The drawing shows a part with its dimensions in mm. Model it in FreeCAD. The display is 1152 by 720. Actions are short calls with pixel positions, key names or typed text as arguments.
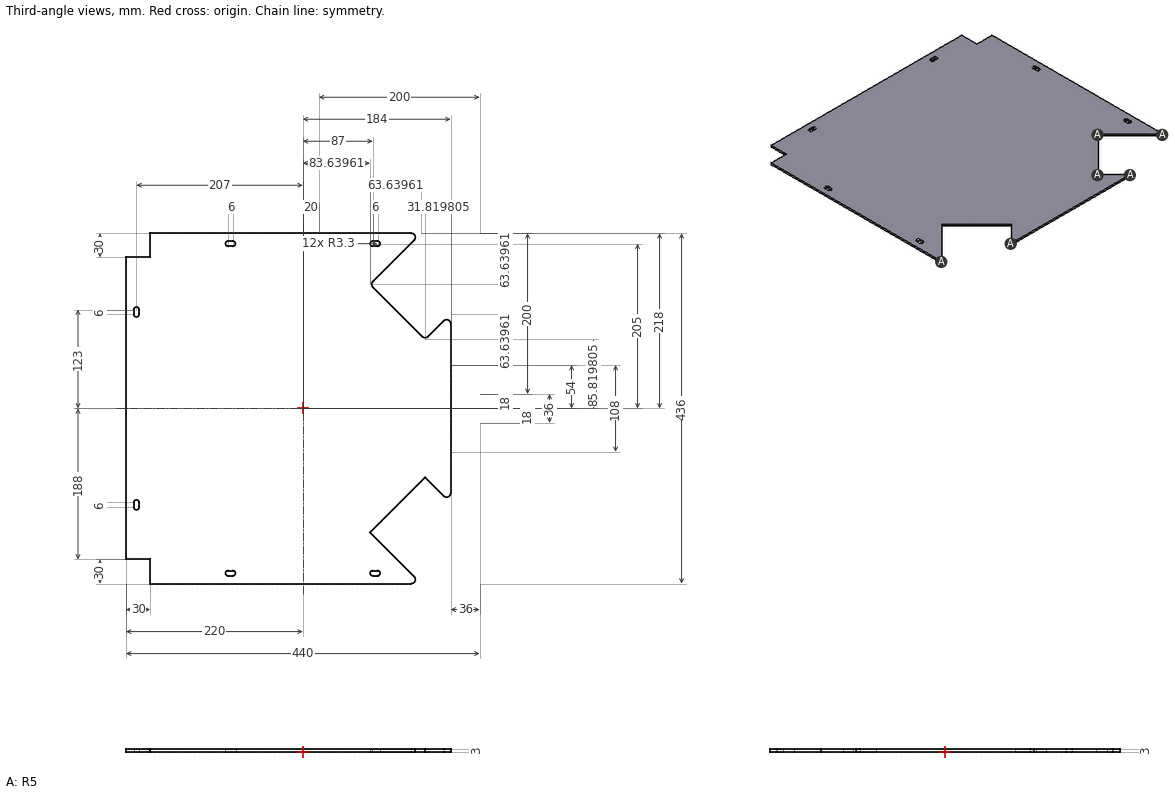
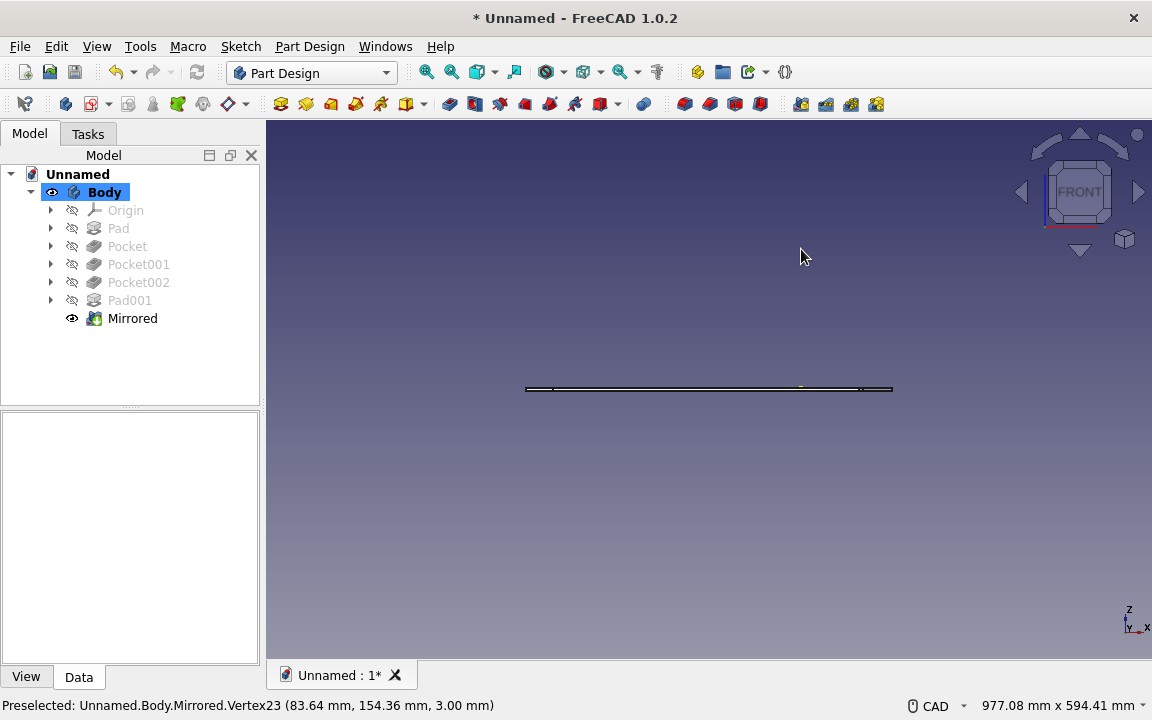
key(v)
key(f)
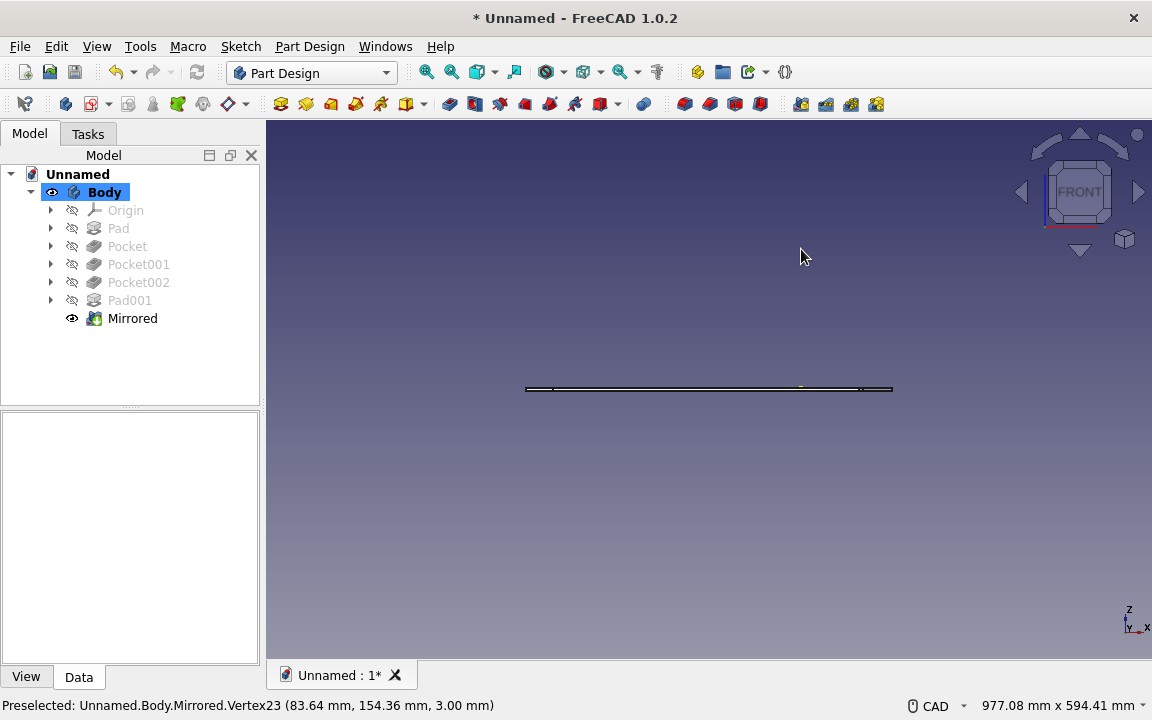
scroll(801, 389, up, 14)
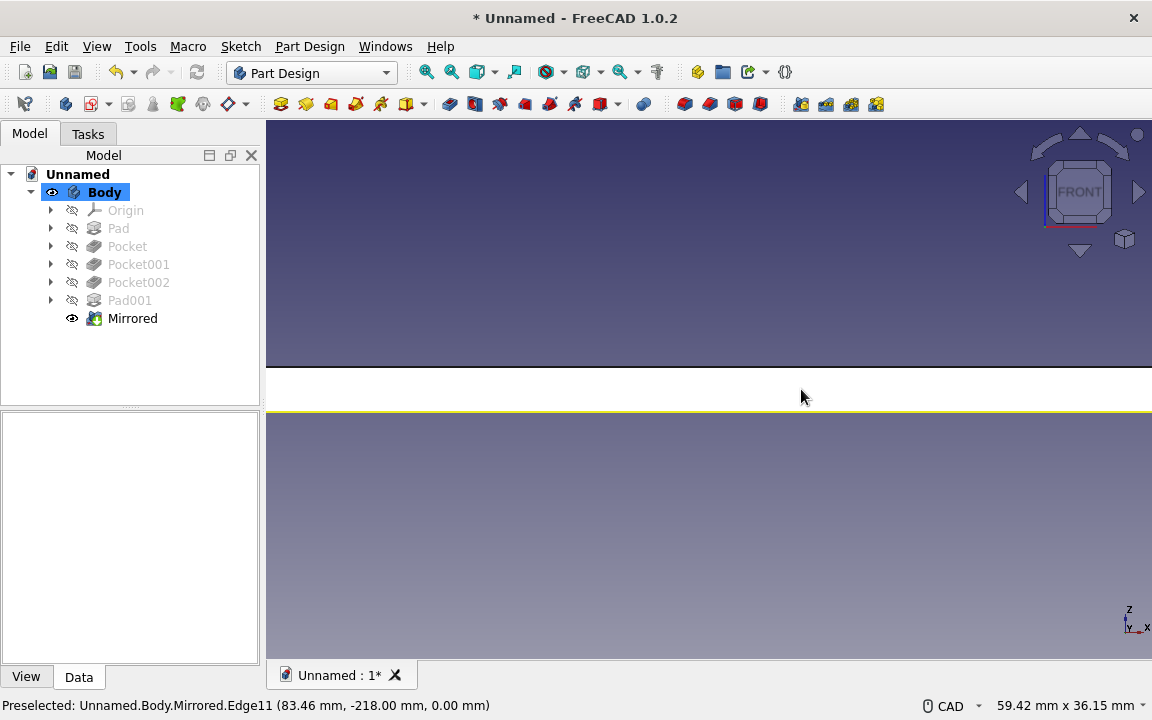
click(427, 72)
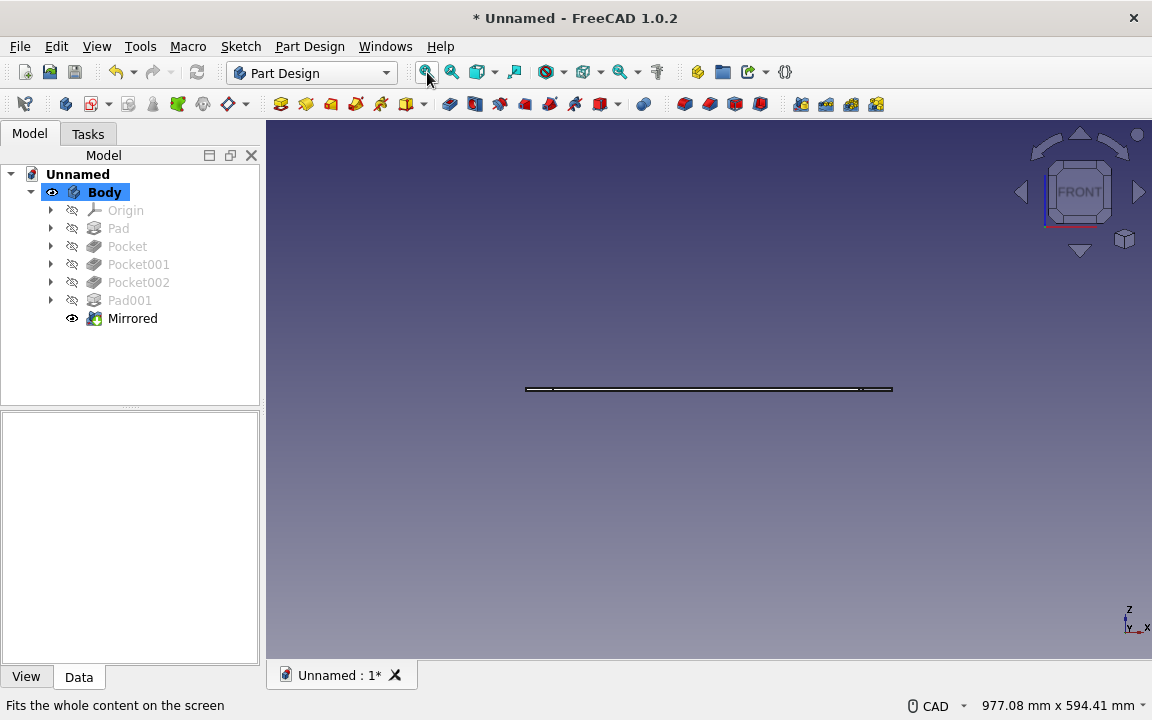
key(3)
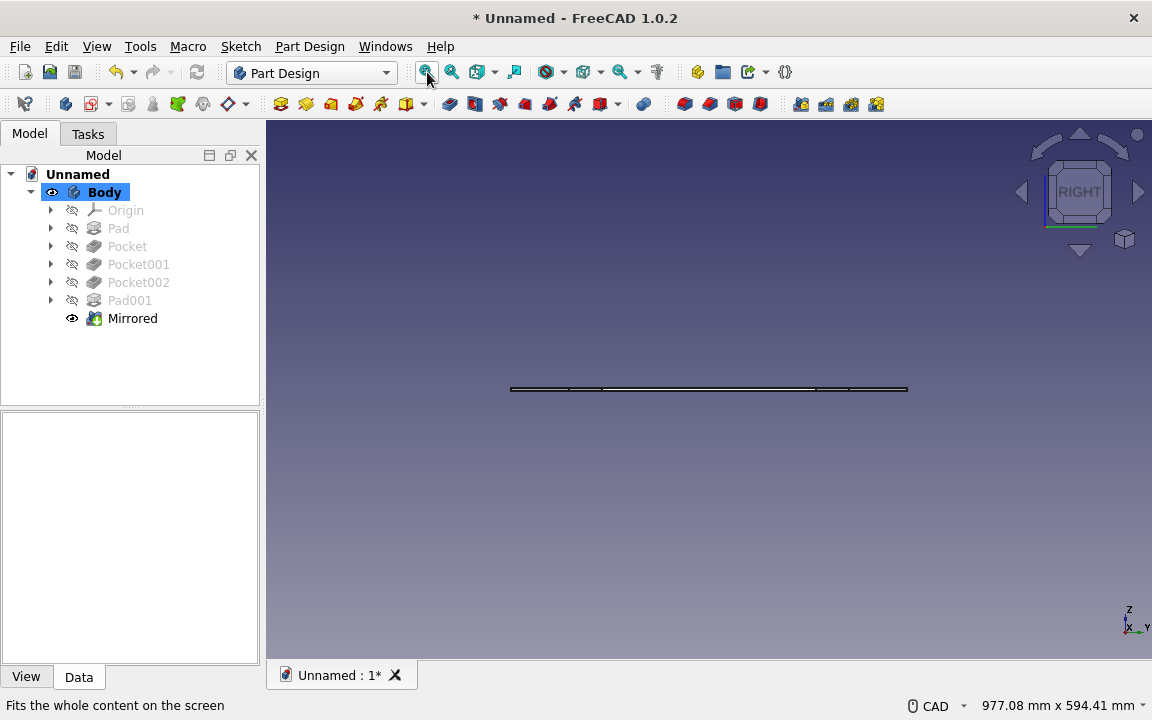
key(v)
key(f)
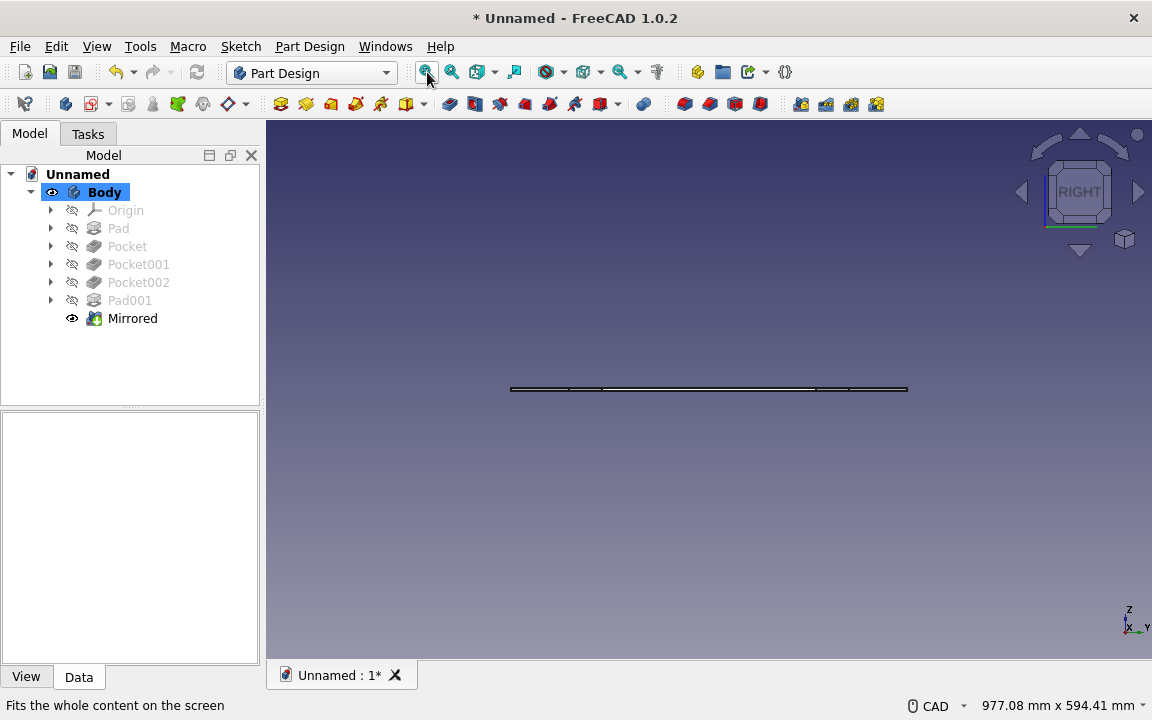
scroll(849, 388, up, 14)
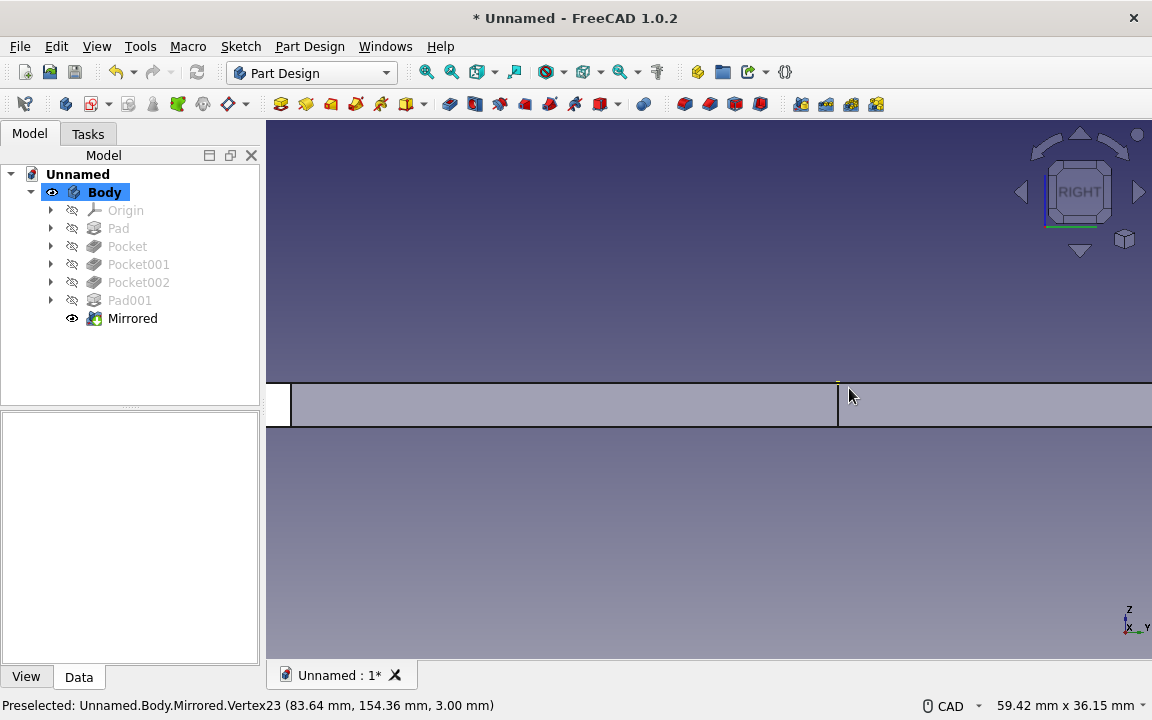
click(427, 72)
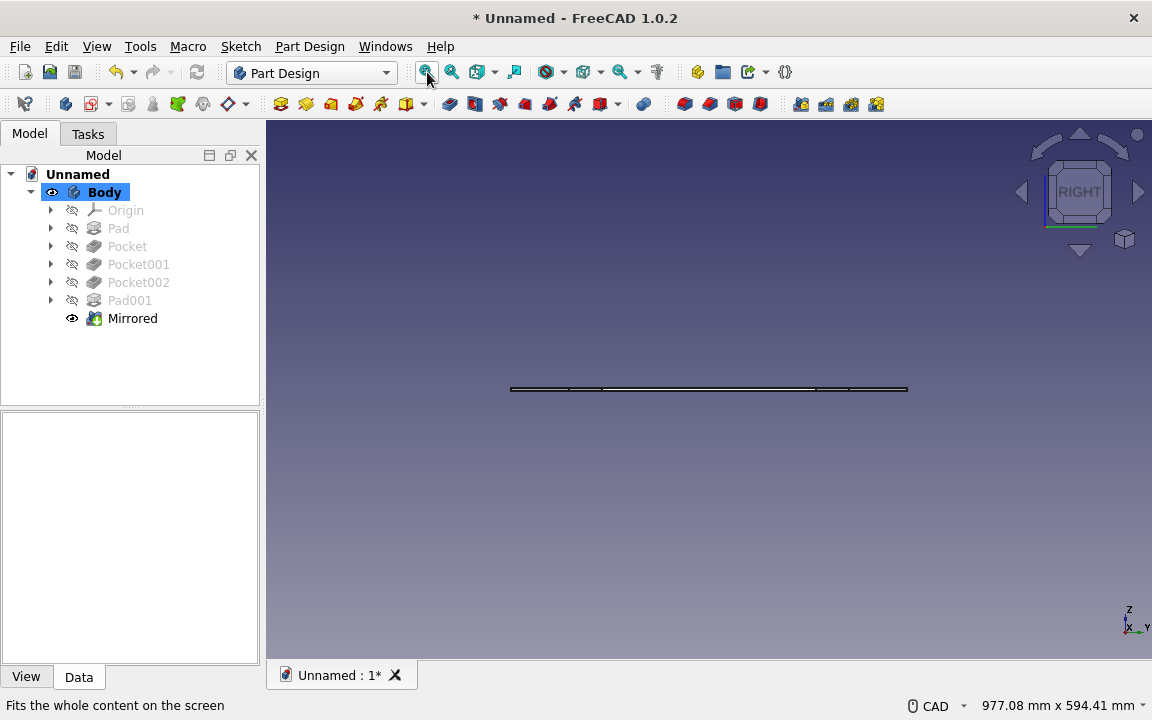
key(5)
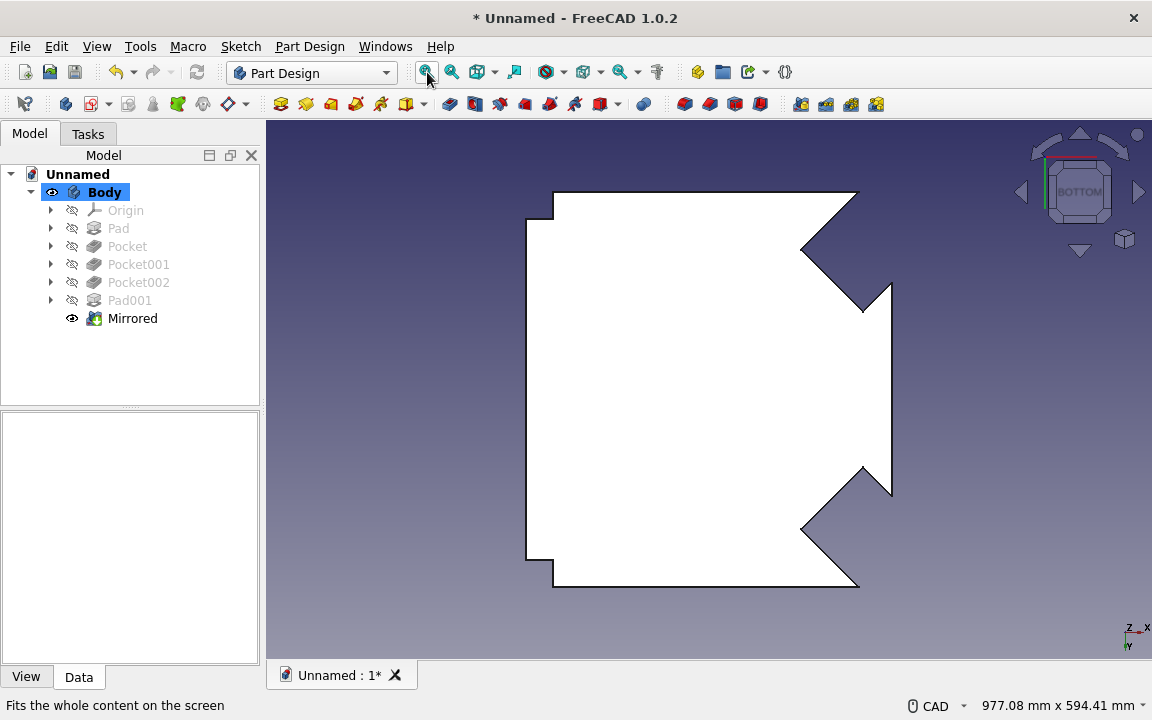
scroll(801, 528, up, 14)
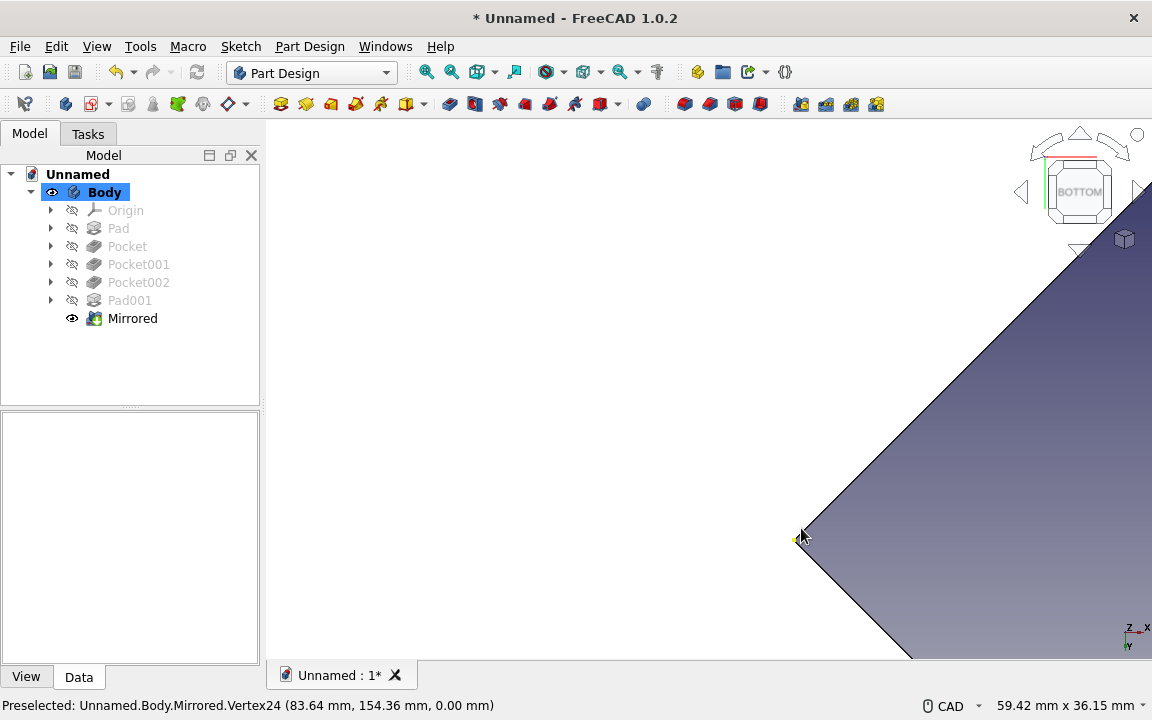
key(v)
key(f)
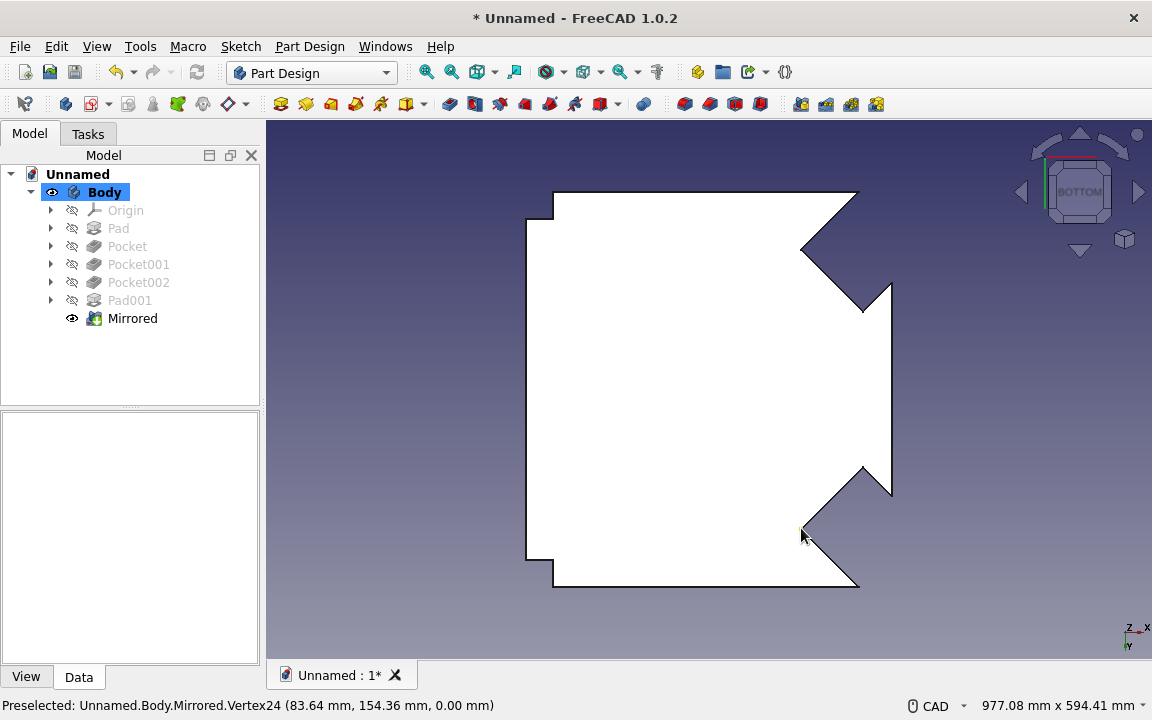
key(4)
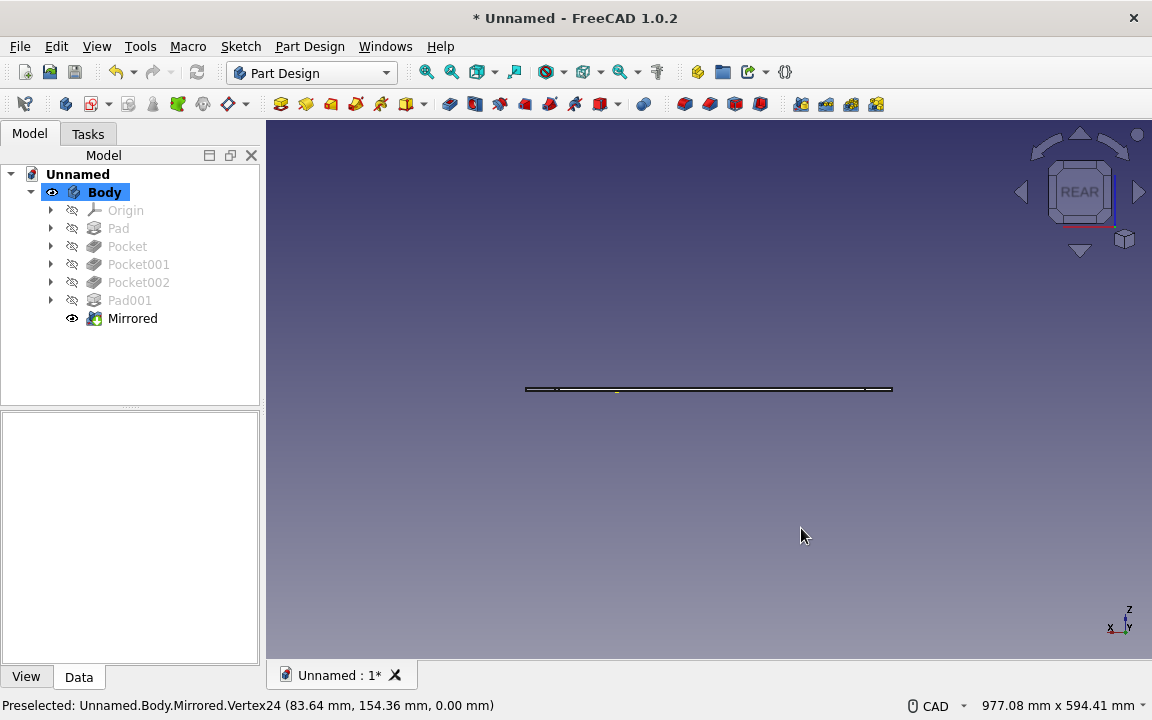
key(v)
key(f)